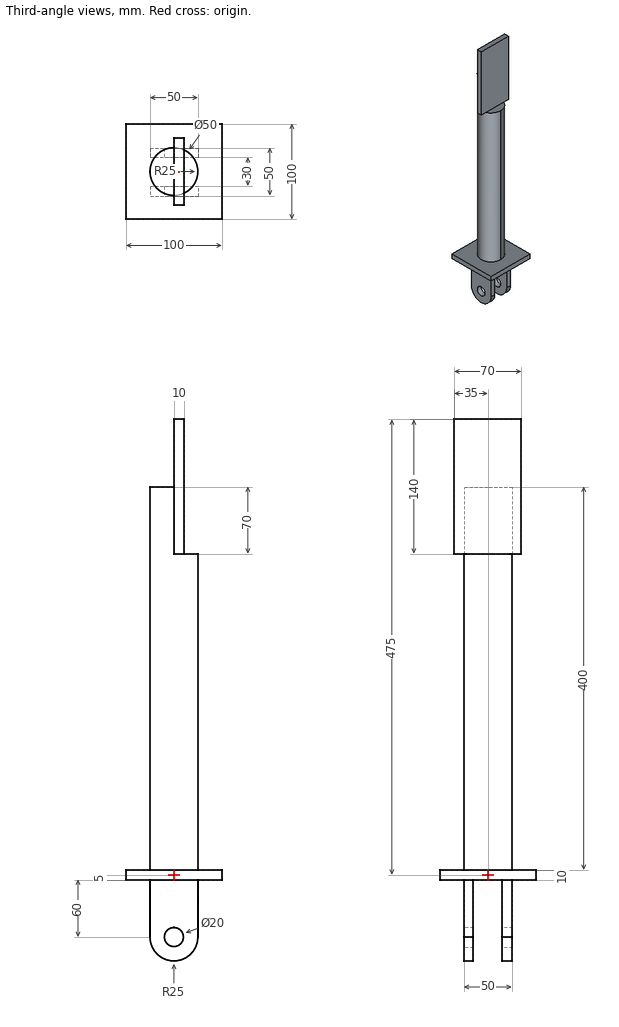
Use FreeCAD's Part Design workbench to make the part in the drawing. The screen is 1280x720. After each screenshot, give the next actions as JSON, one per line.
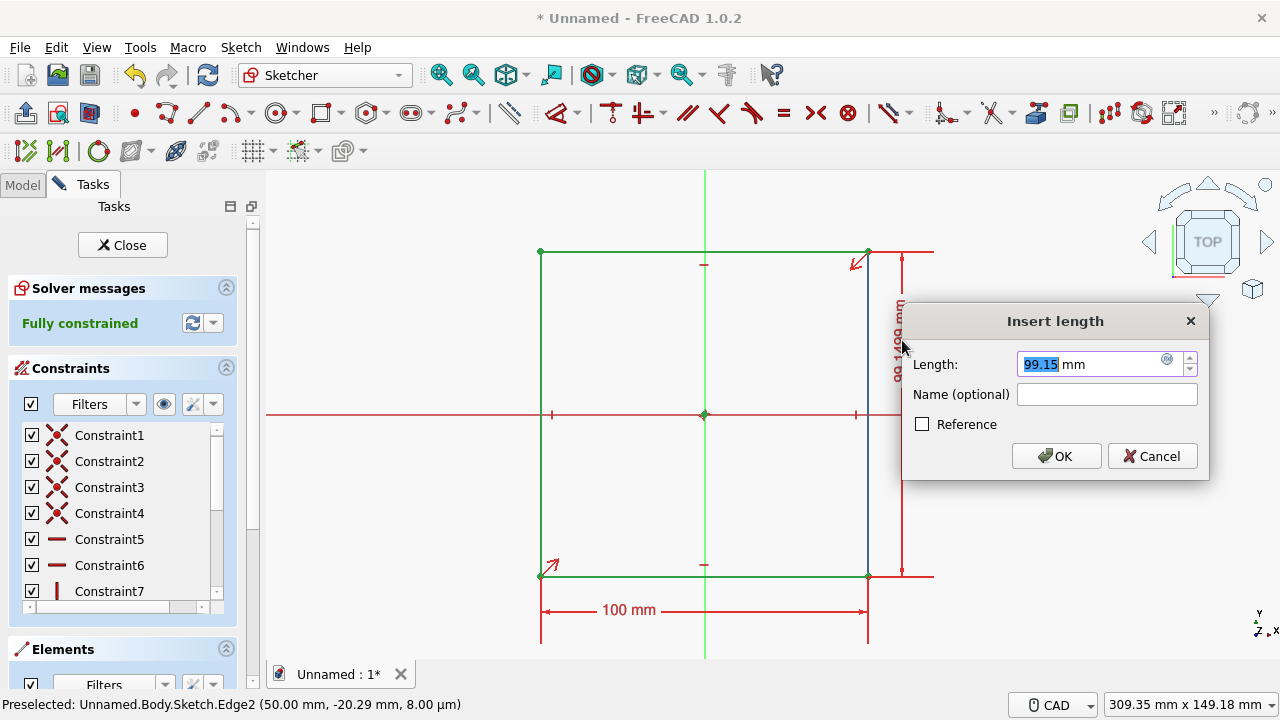
{"action": "type", "text": "100"}
{"action": "key", "text": "Return"}
{"action": "key", "text": "Escape"}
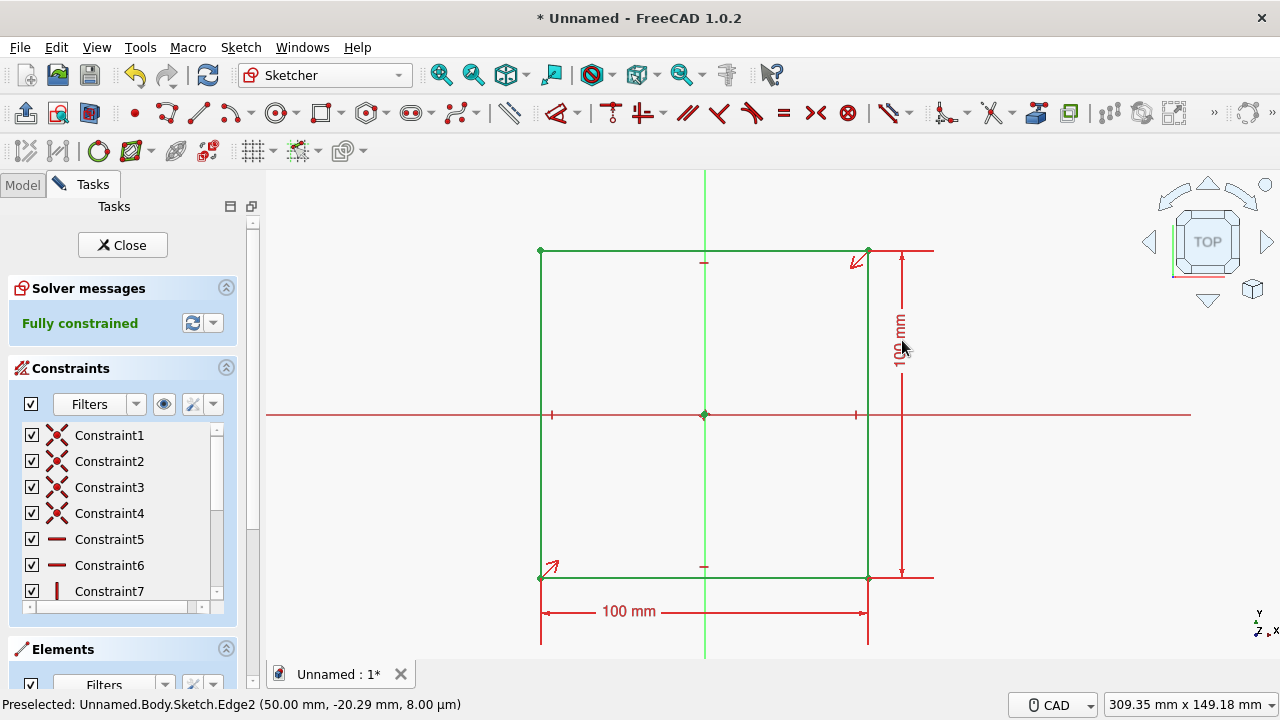
{"action": "left_click", "coordinate": [123, 245]}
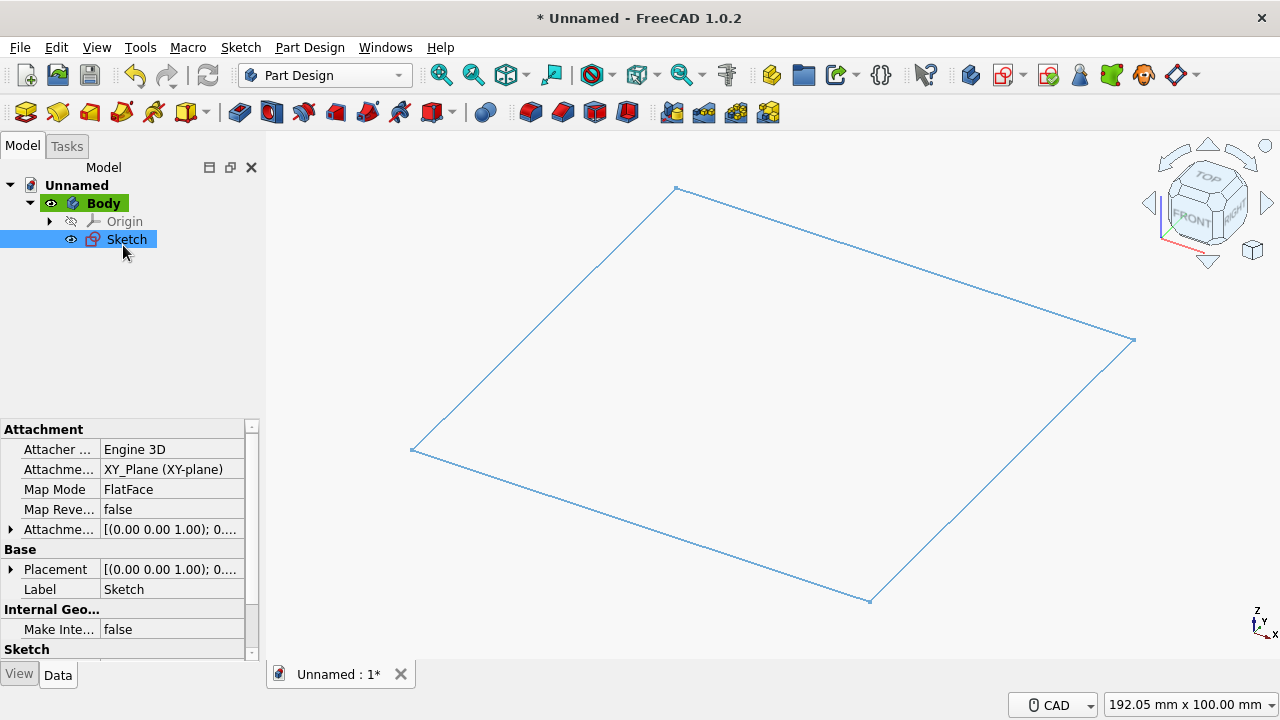
{"action": "left_click", "coordinate": [26, 112]}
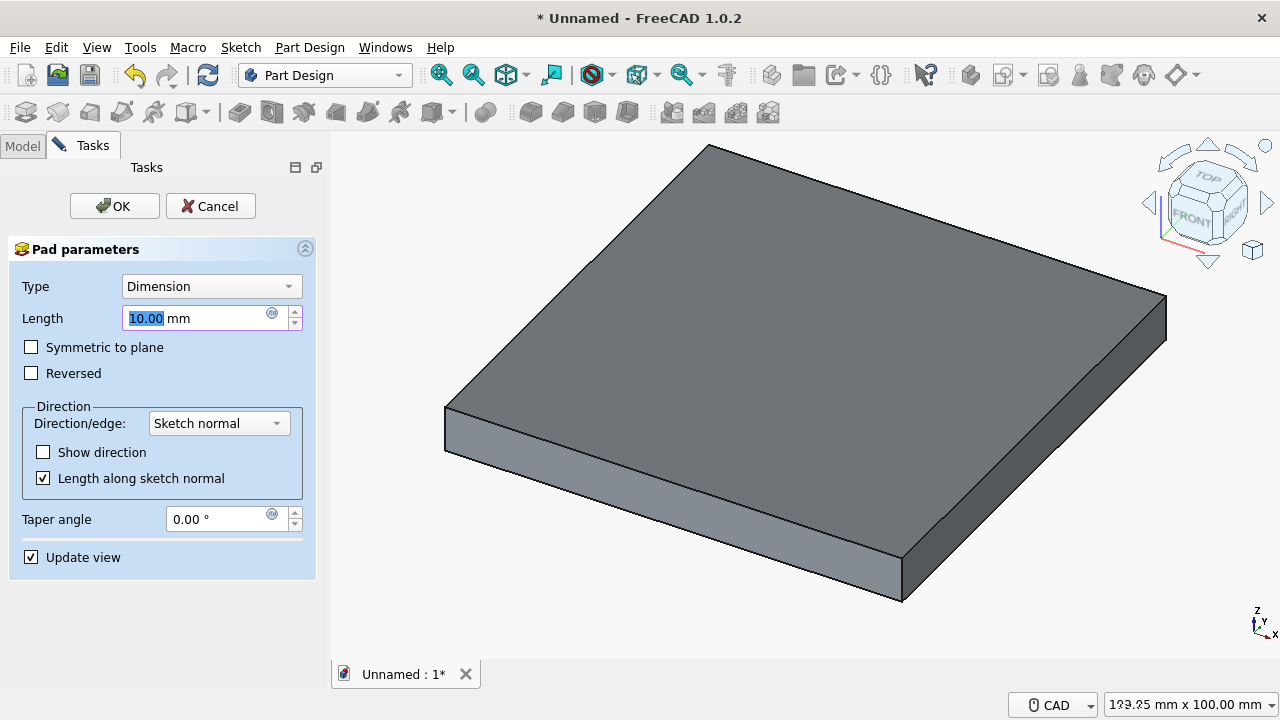
{"action": "type", "text": "10"}
{"action": "key", "text": "Tab"}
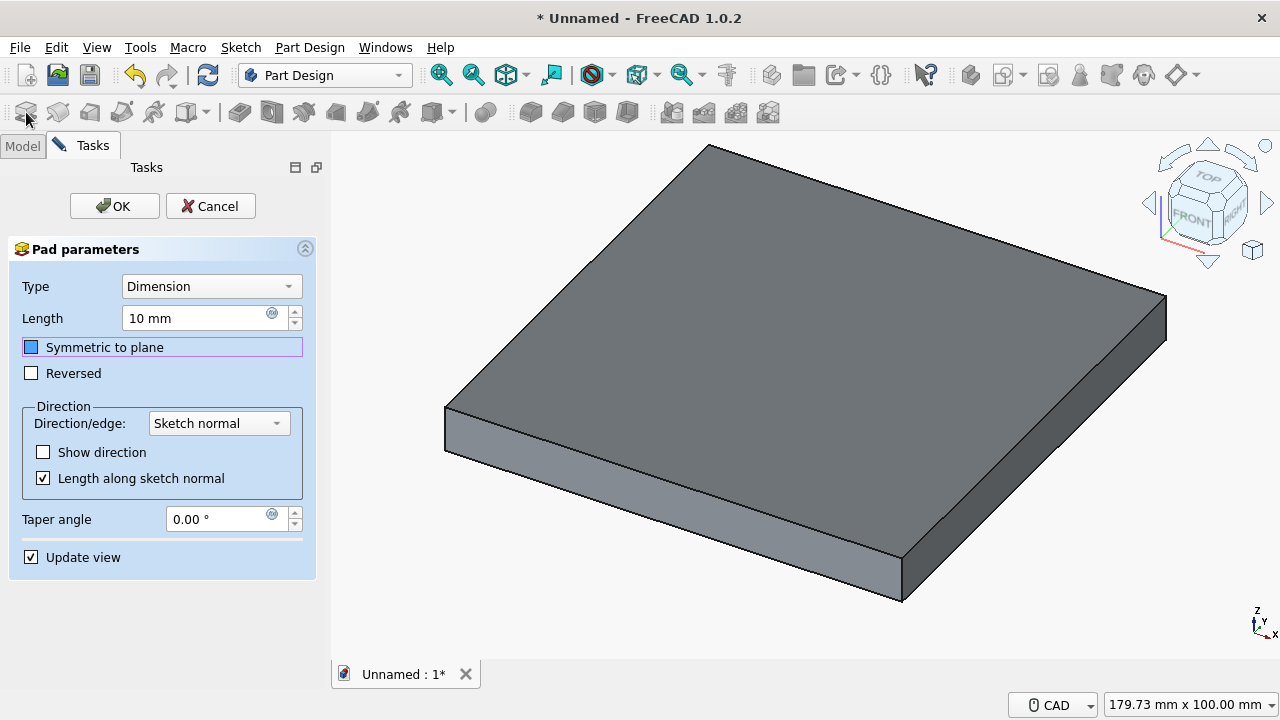
{"action": "left_click", "coordinate": [30, 347]}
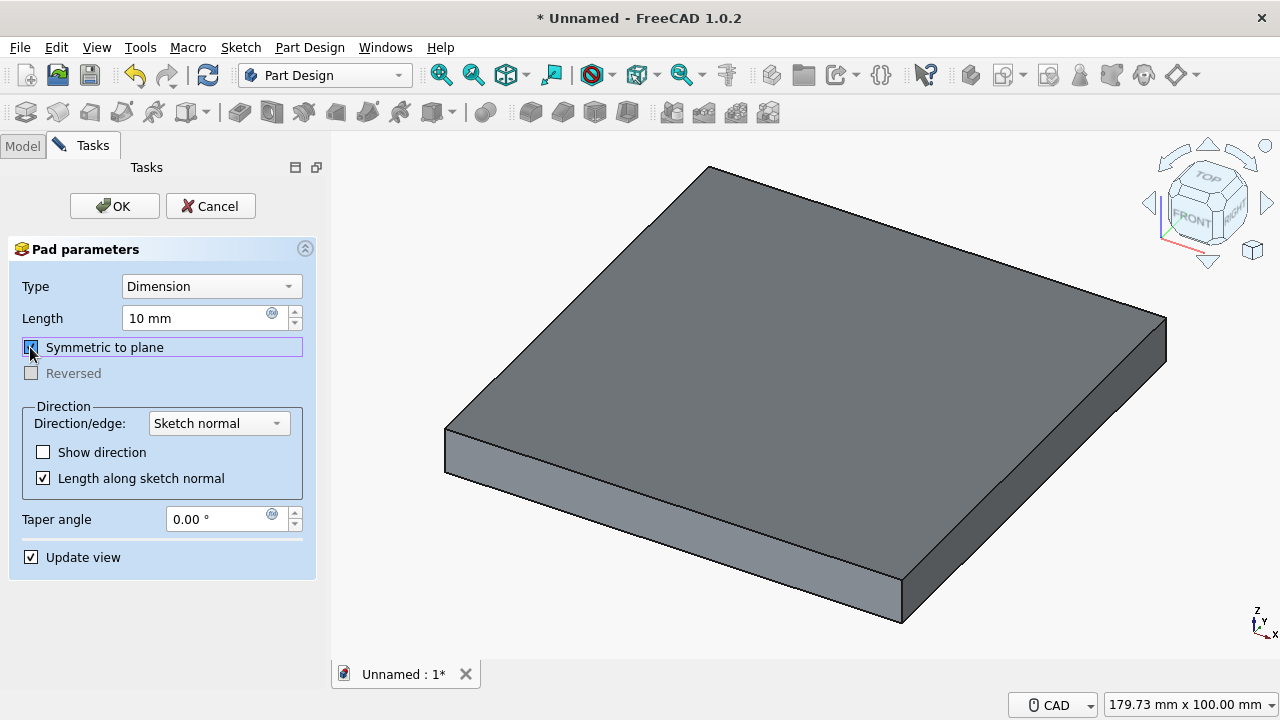
{"action": "left_click", "coordinate": [115, 206]}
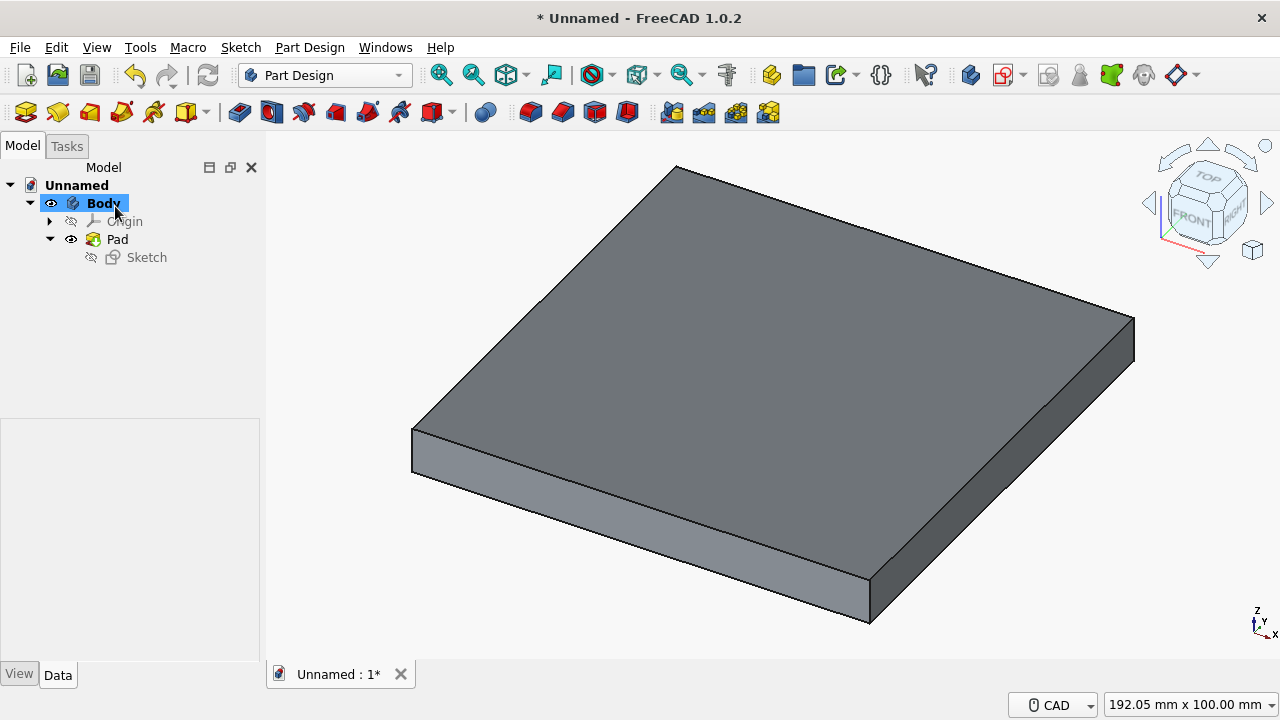
{"action": "left_click", "coordinate": [1004, 76]}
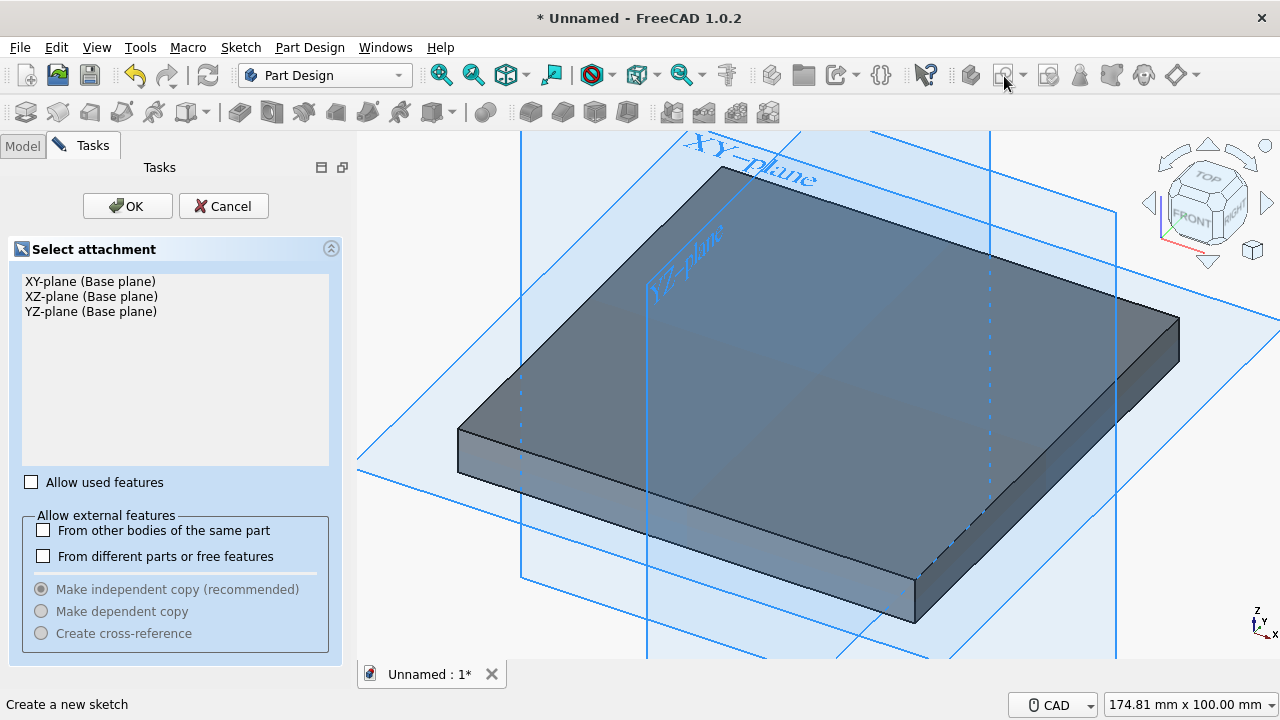
{"action": "left_click", "coordinate": [82, 296]}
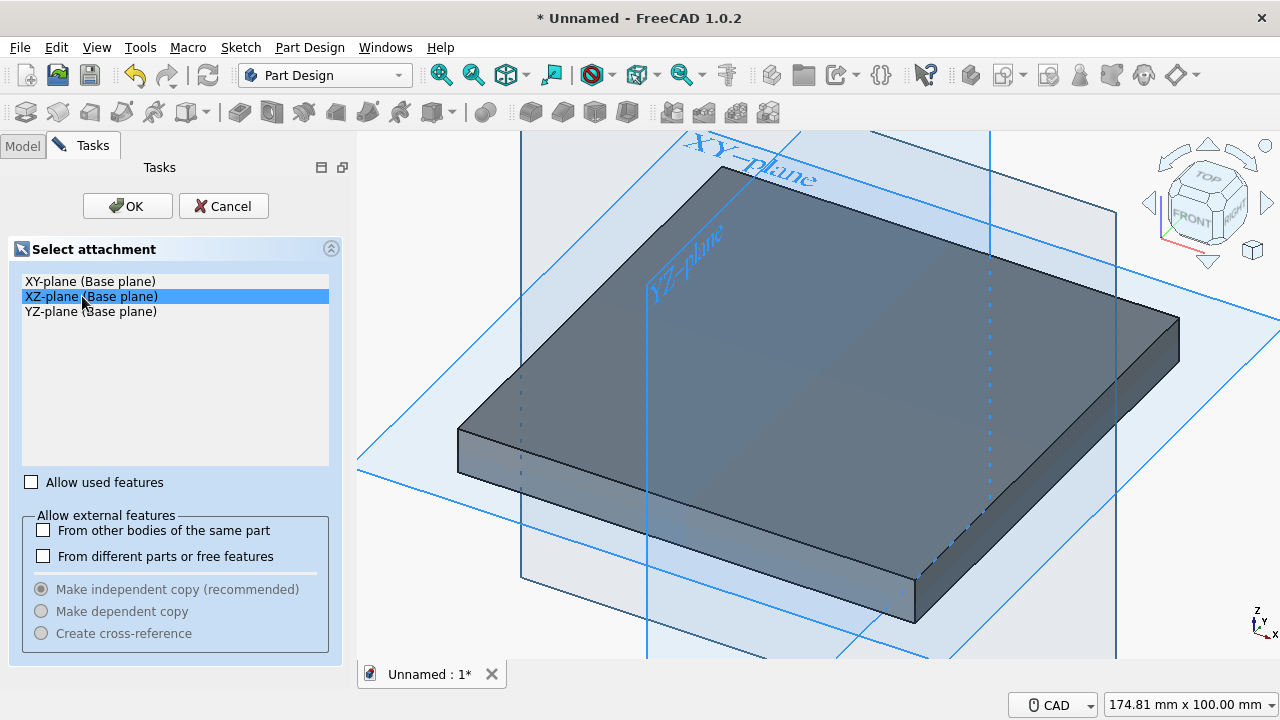
{"action": "left_click", "coordinate": [128, 206]}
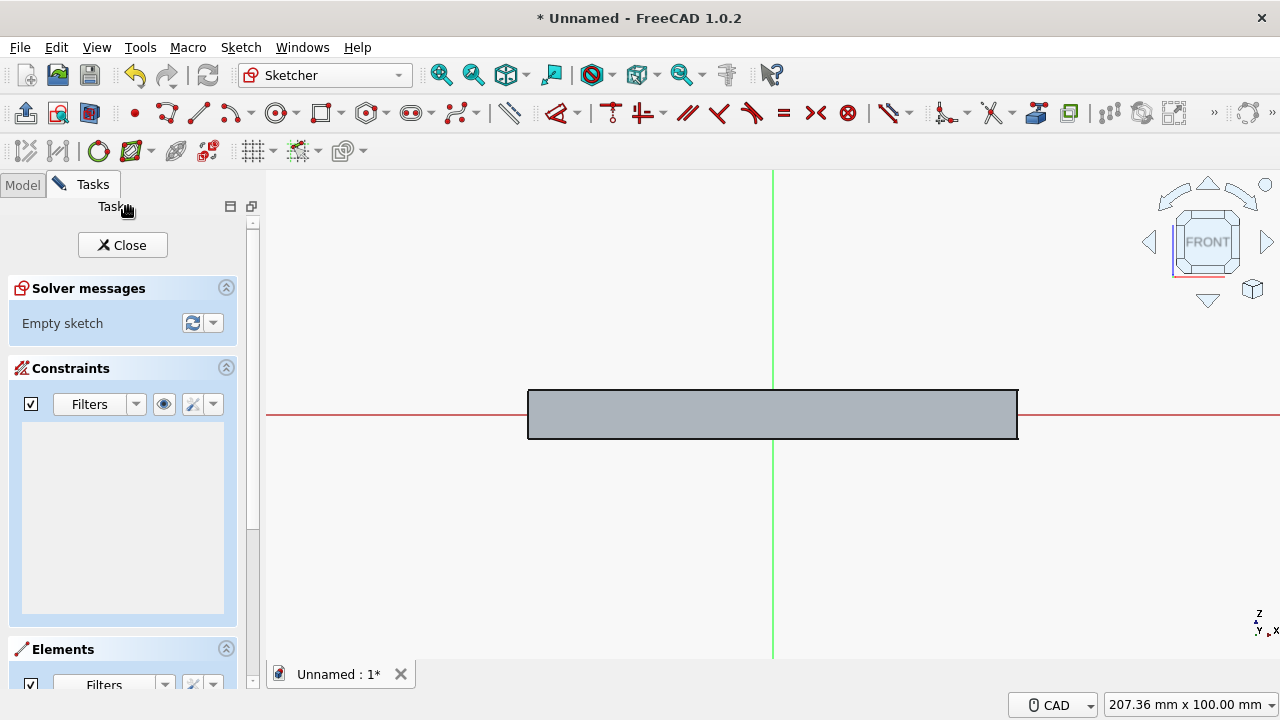
{"action": "key", "text": "q s"}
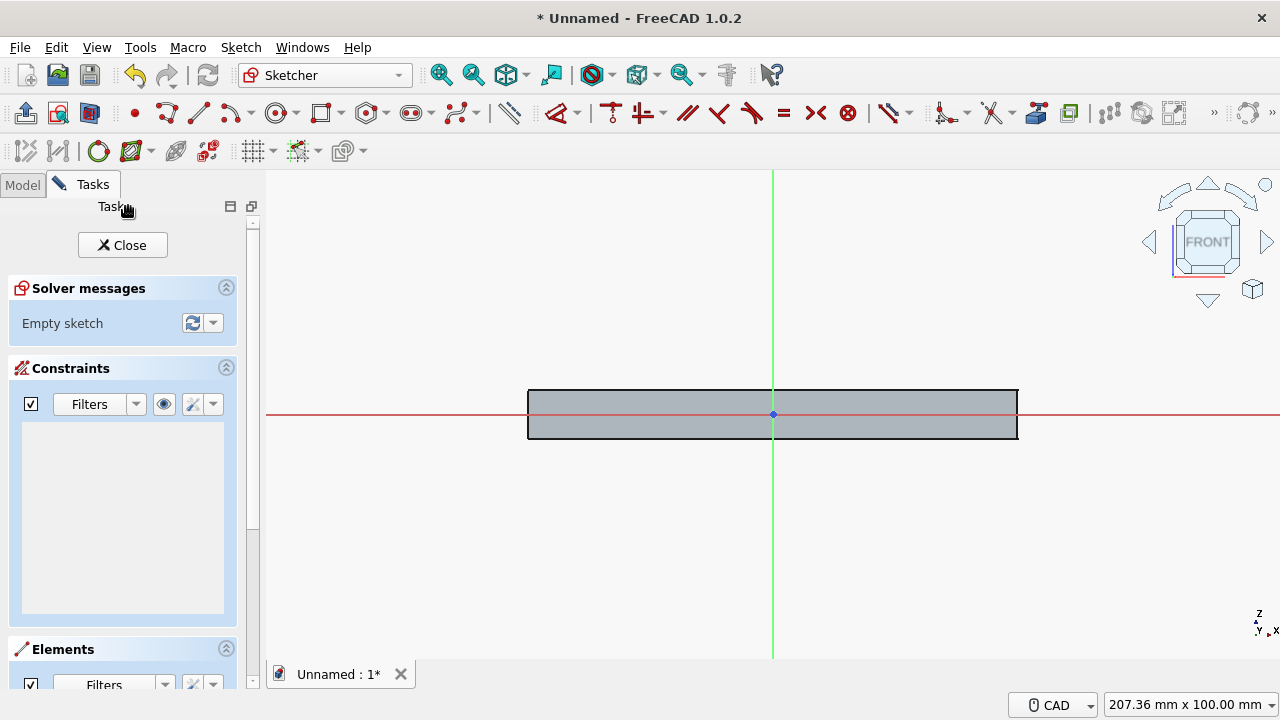
{"action": "scroll", "coordinate": [621, 198], "scroll_direction": "down", "scroll_amount": 3}